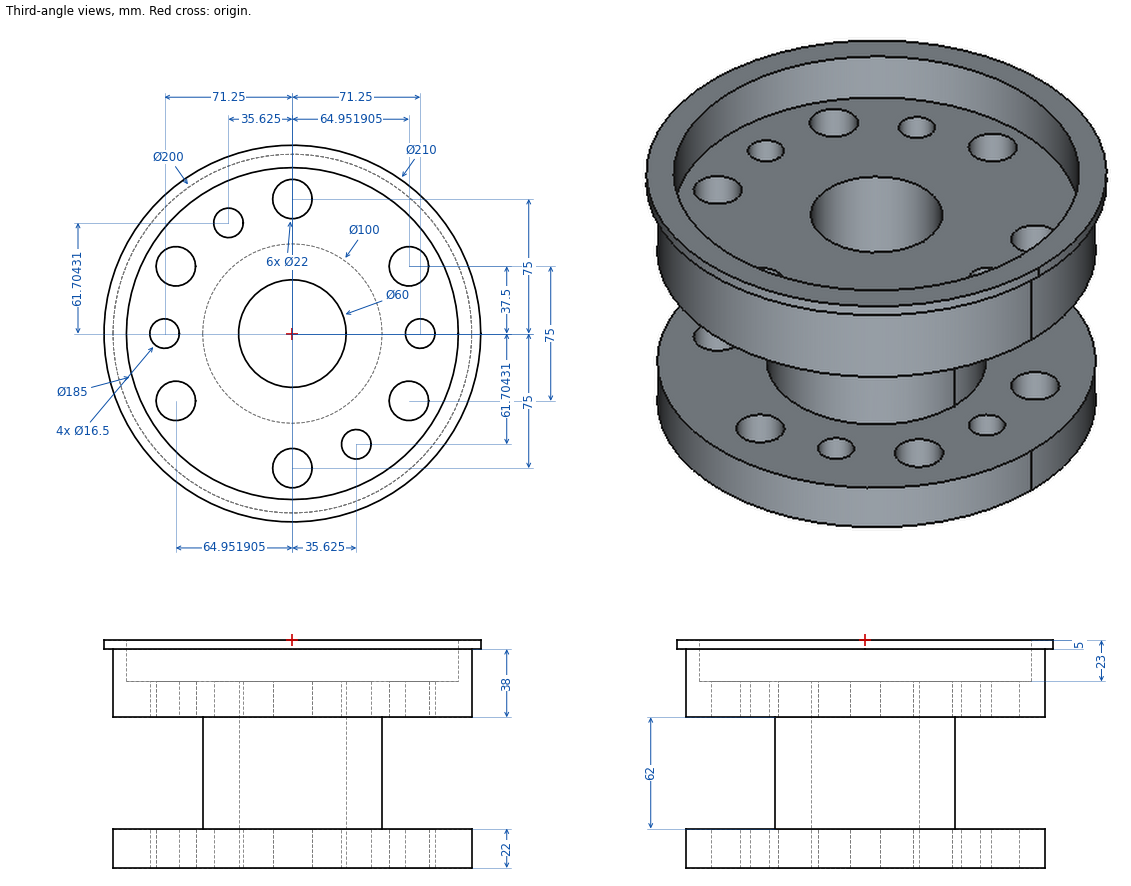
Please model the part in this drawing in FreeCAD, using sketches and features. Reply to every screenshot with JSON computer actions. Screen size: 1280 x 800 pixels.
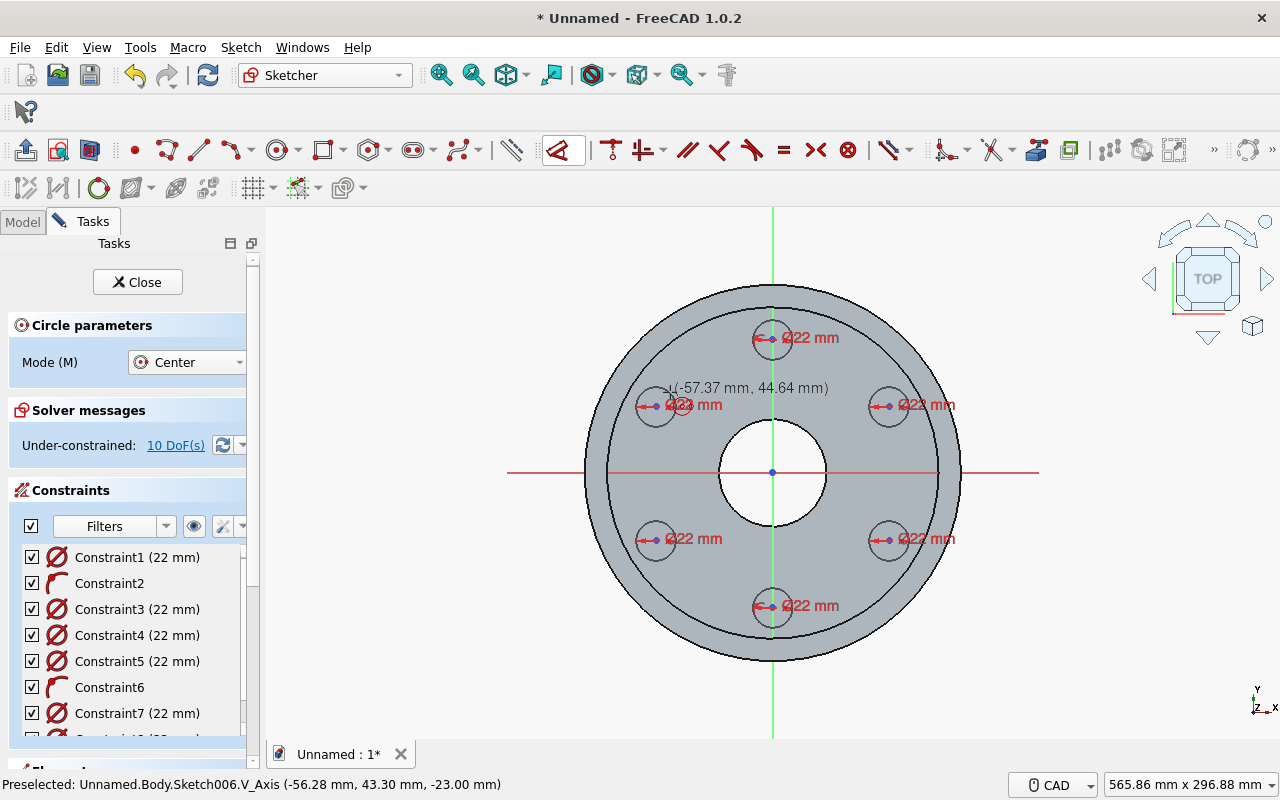
{"action": "scroll", "coordinate": [645, 473], "scroll_direction": "up", "scroll_amount": 3}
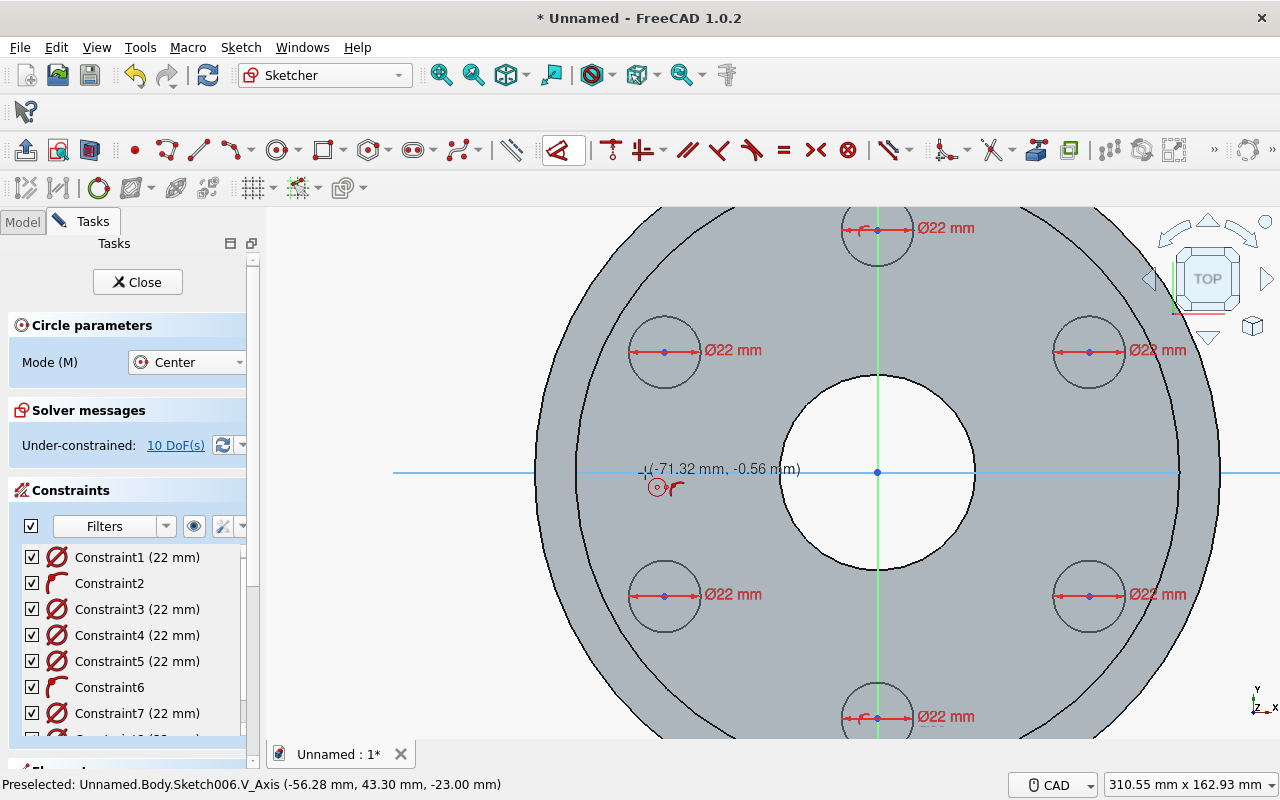
{"action": "left_click", "coordinate": [645, 473]}
{"action": "mouse_move", "coordinate": [664, 454]}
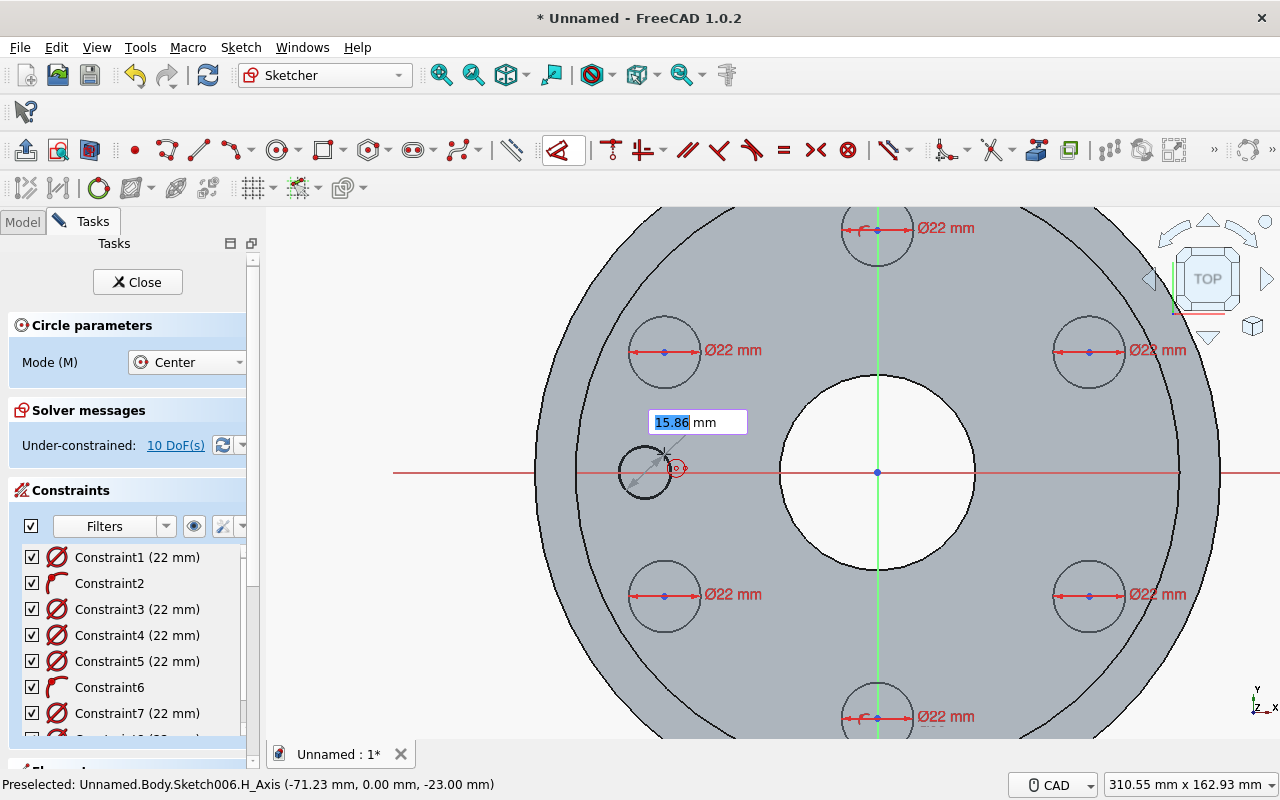
{"action": "type", "text": "16.5"}
{"action": "key", "text": "Return"}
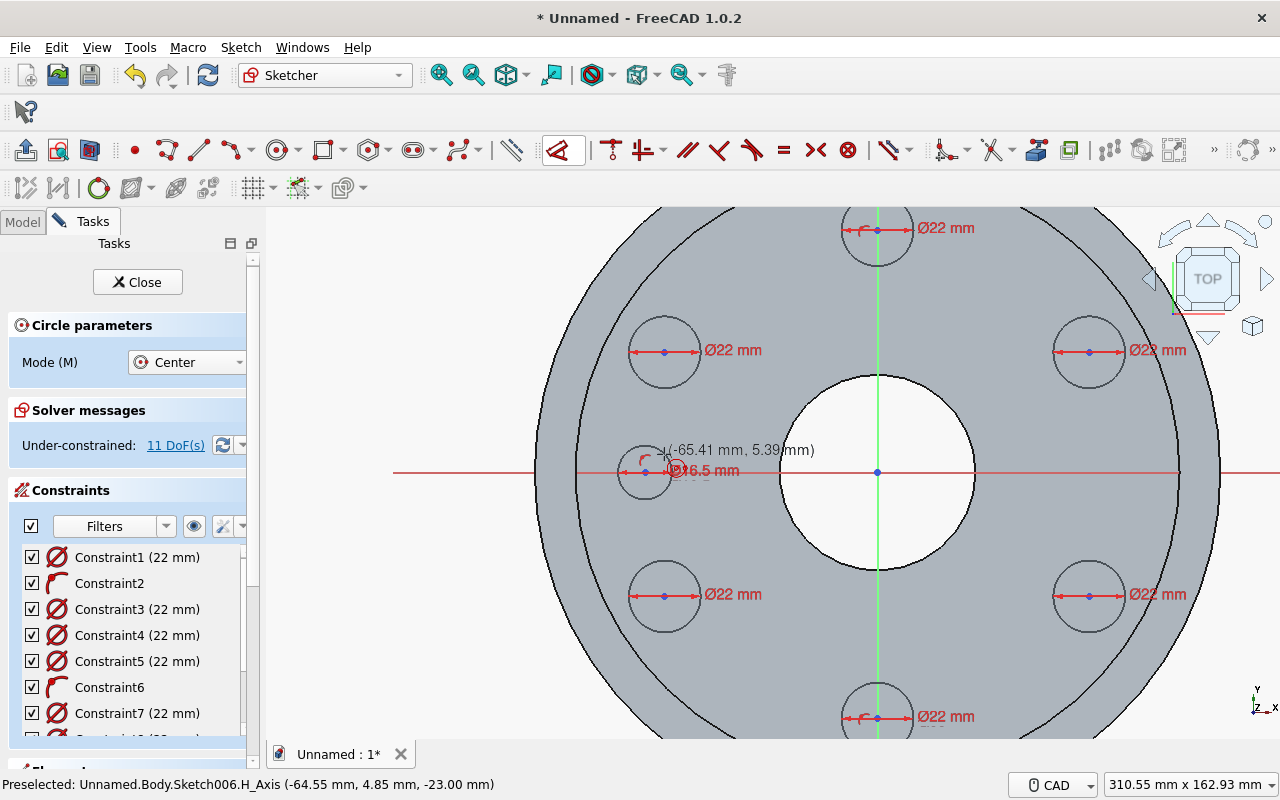
{"action": "left_click", "coordinate": [1110, 473]}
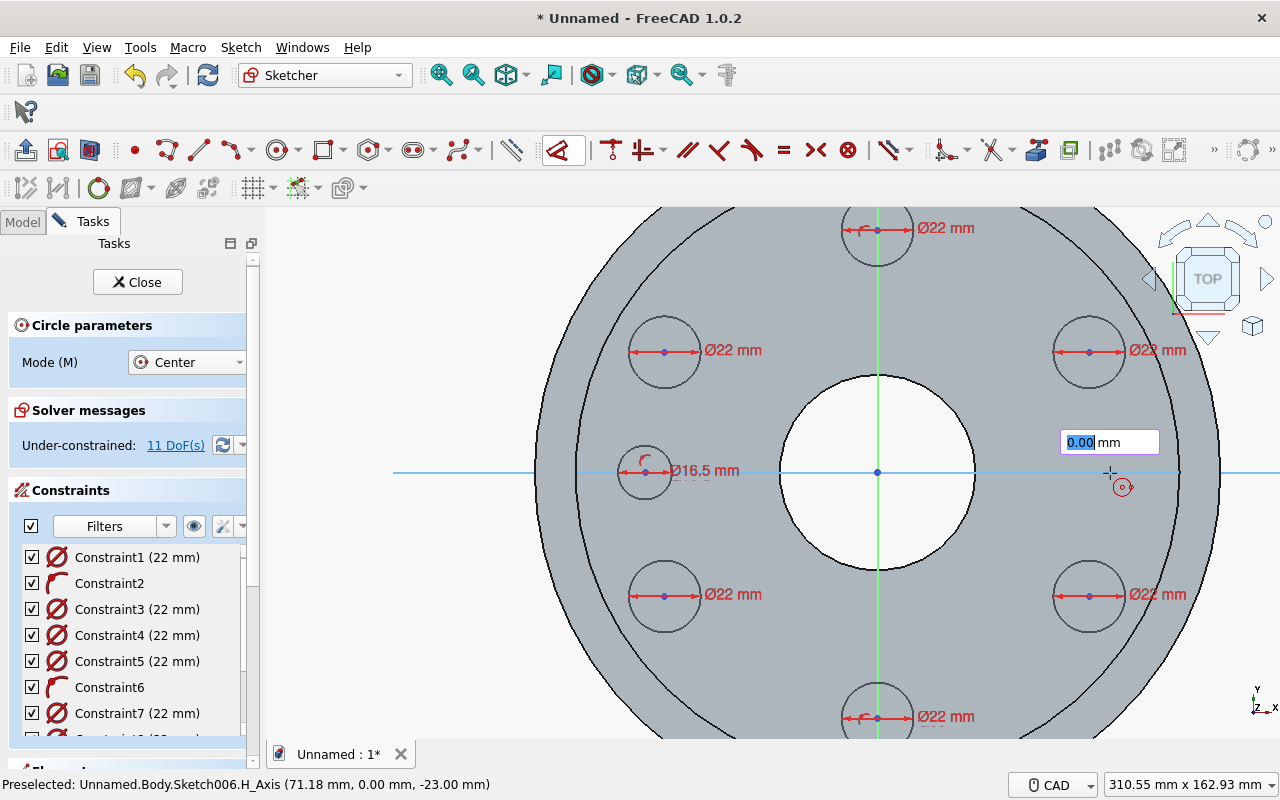
{"action": "scroll", "coordinate": [494, 474], "scroll_direction": "down", "scroll_amount": 3}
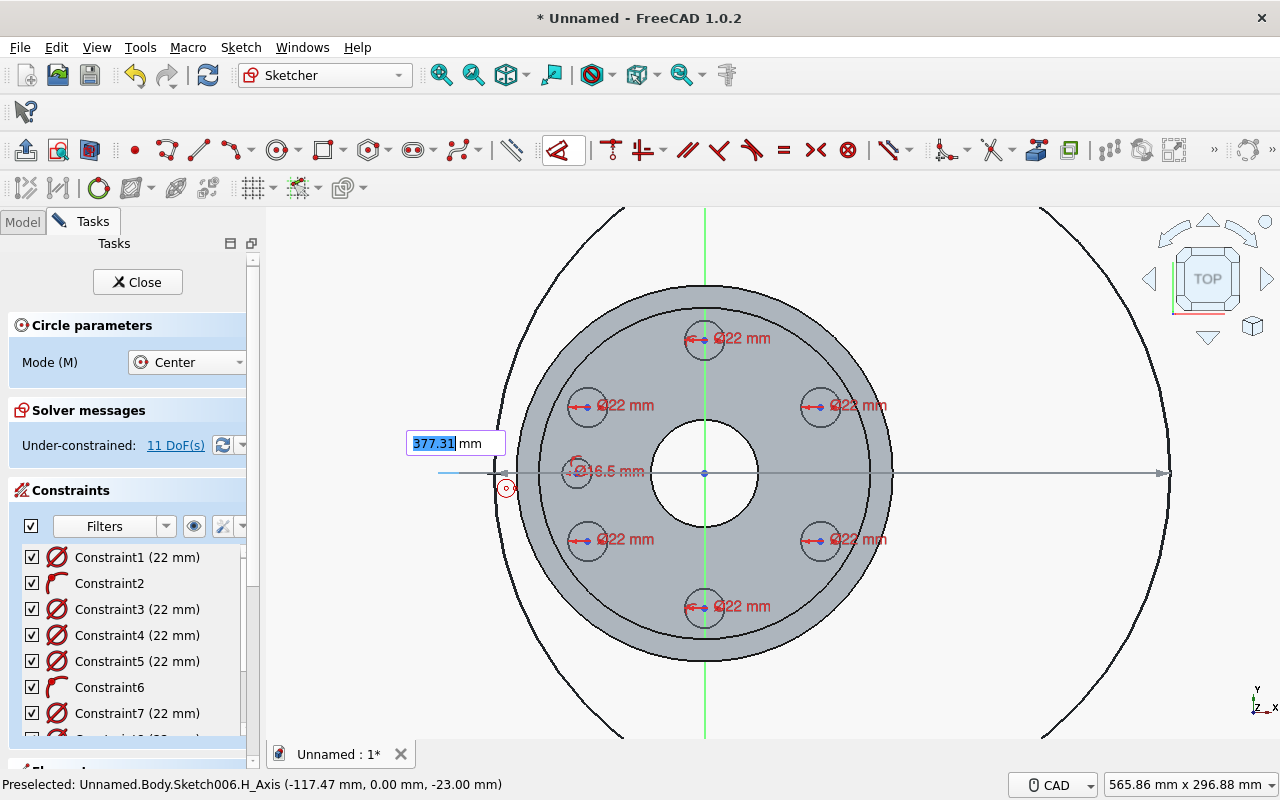
{"action": "scroll", "coordinate": [843, 463], "scroll_direction": "up", "scroll_amount": 3}
{"action": "mouse_move", "coordinate": [842, 463]}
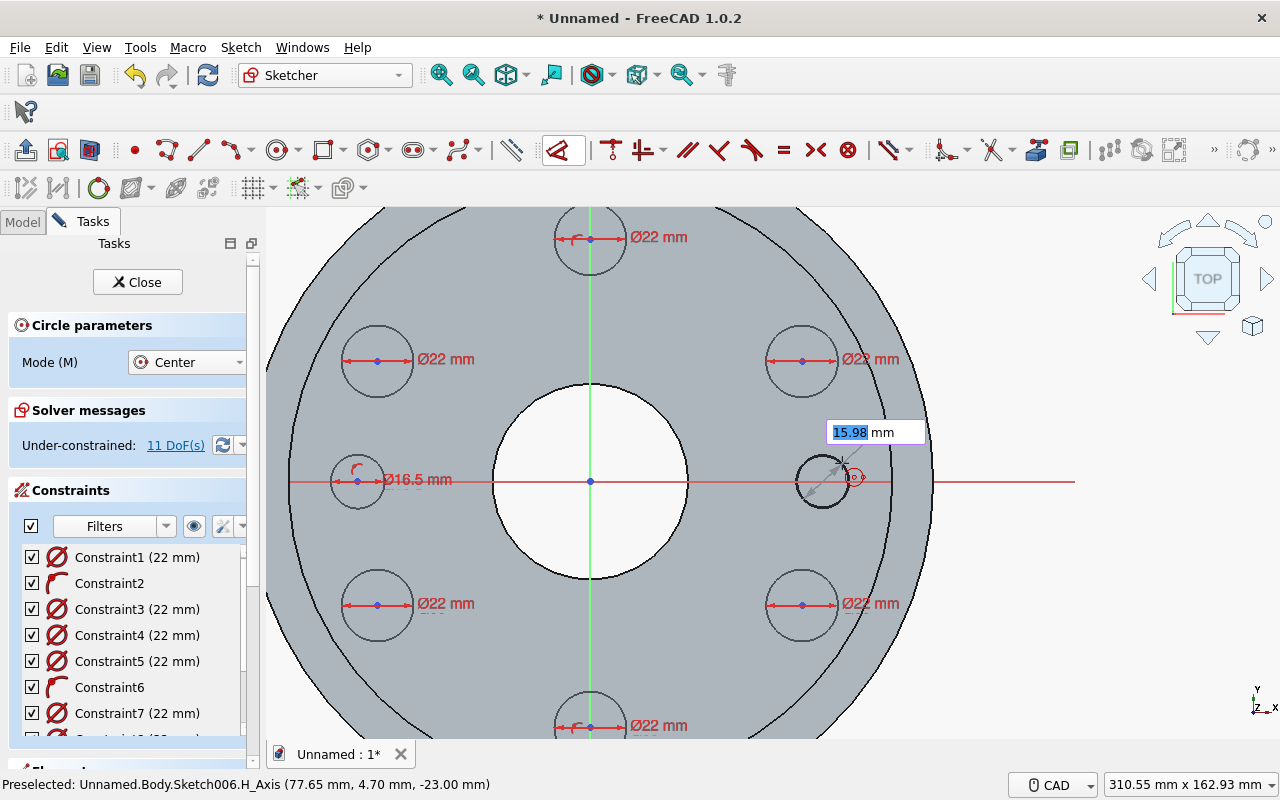
{"action": "type", "text": "16.5"}
{"action": "key", "text": "Return"}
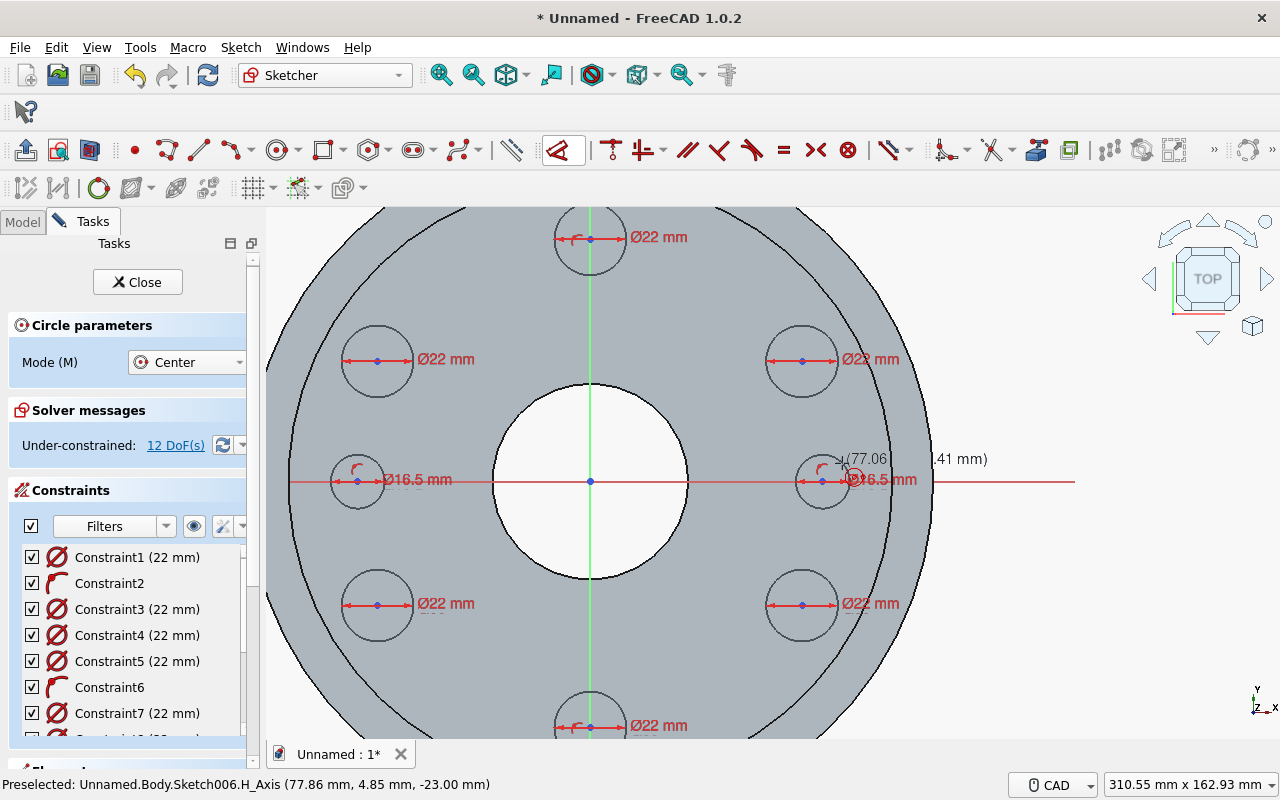
{"action": "left_click", "coordinate": [707, 683]}
{"action": "mouse_move", "coordinate": [726, 664]}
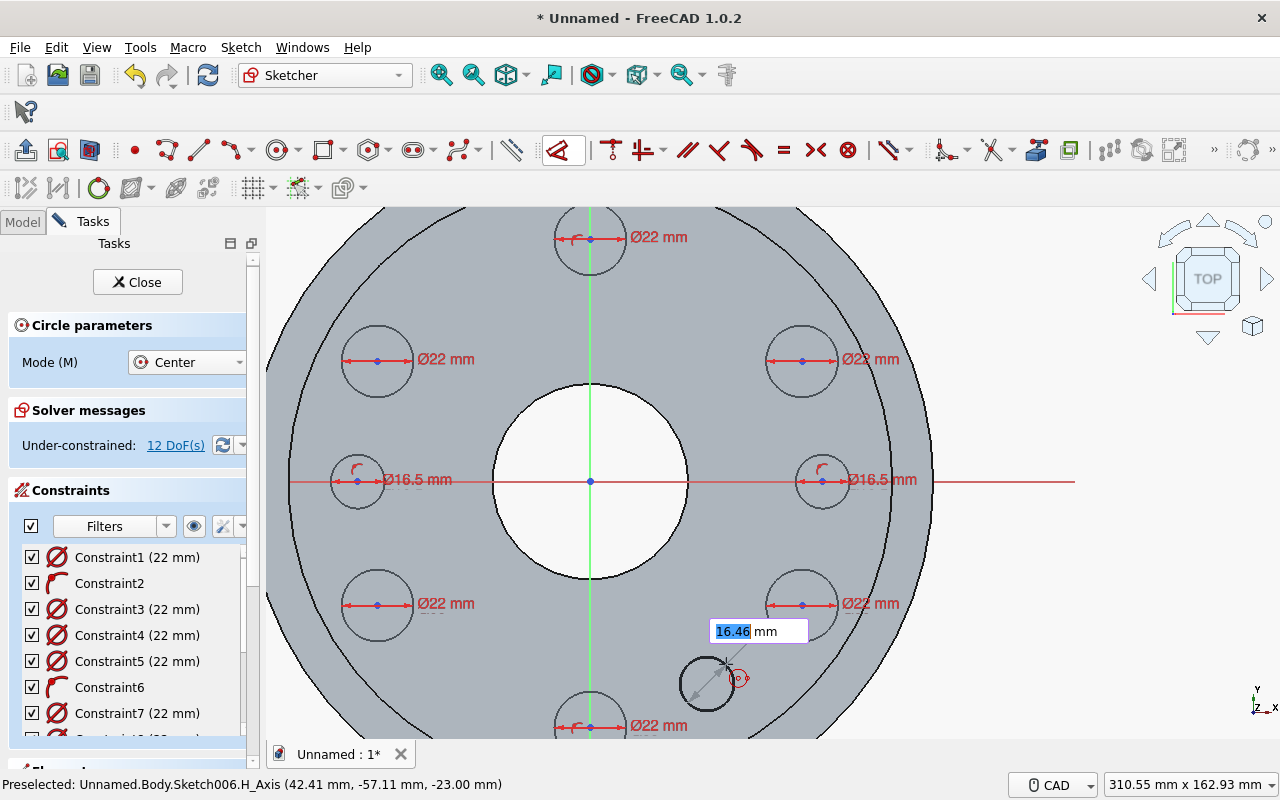
{"action": "type", "text": "16.5"}
{"action": "key", "text": "Return"}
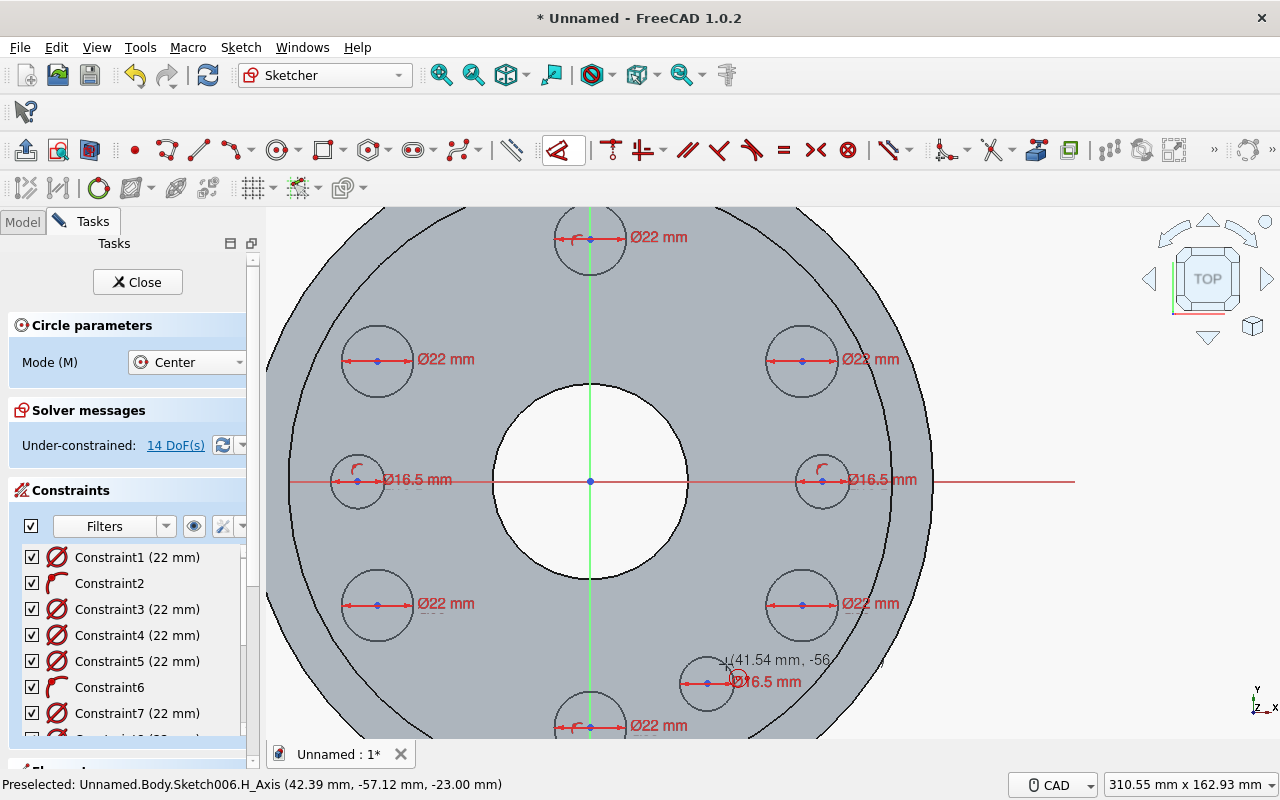
{"action": "left_click", "coordinate": [474, 280]}
{"action": "mouse_move", "coordinate": [493, 261]}